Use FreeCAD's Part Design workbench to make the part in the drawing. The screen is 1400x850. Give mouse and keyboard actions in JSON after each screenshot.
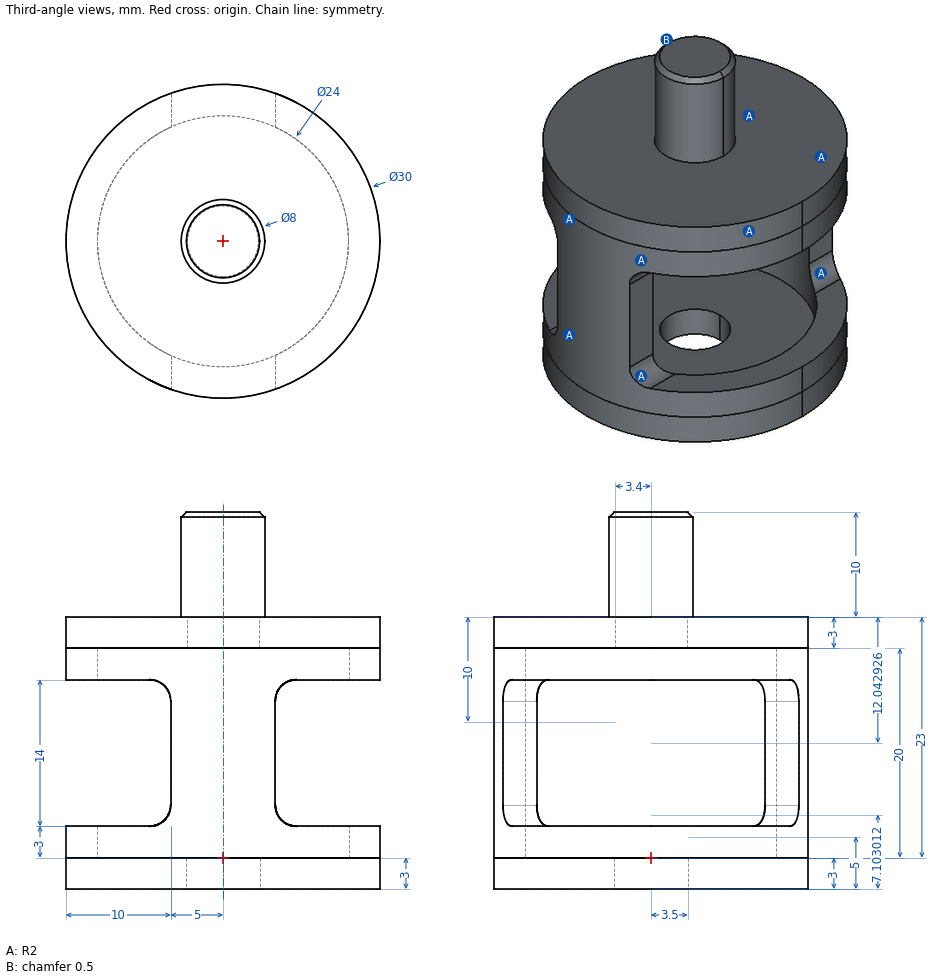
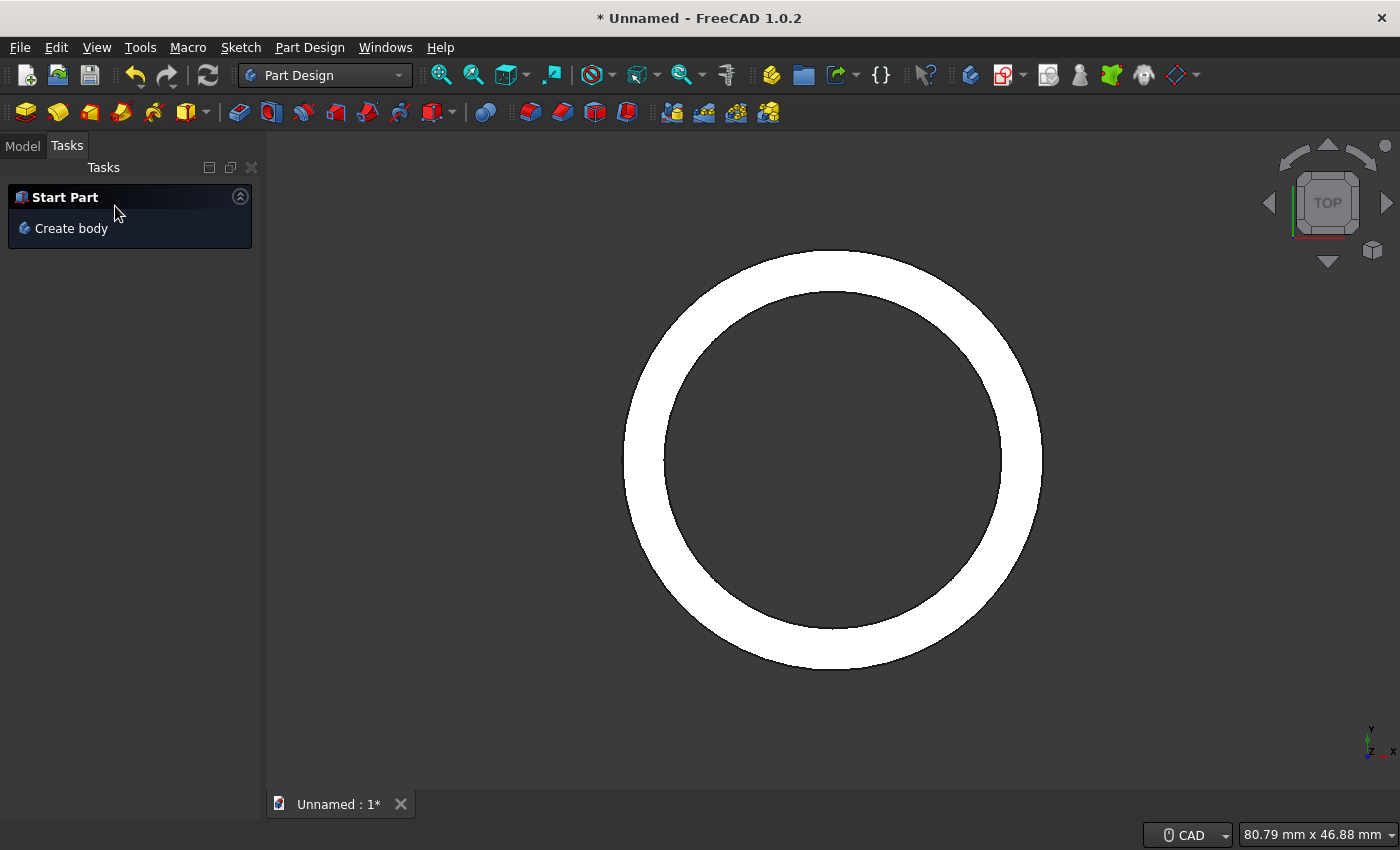
{"action": "key", "text": "1"}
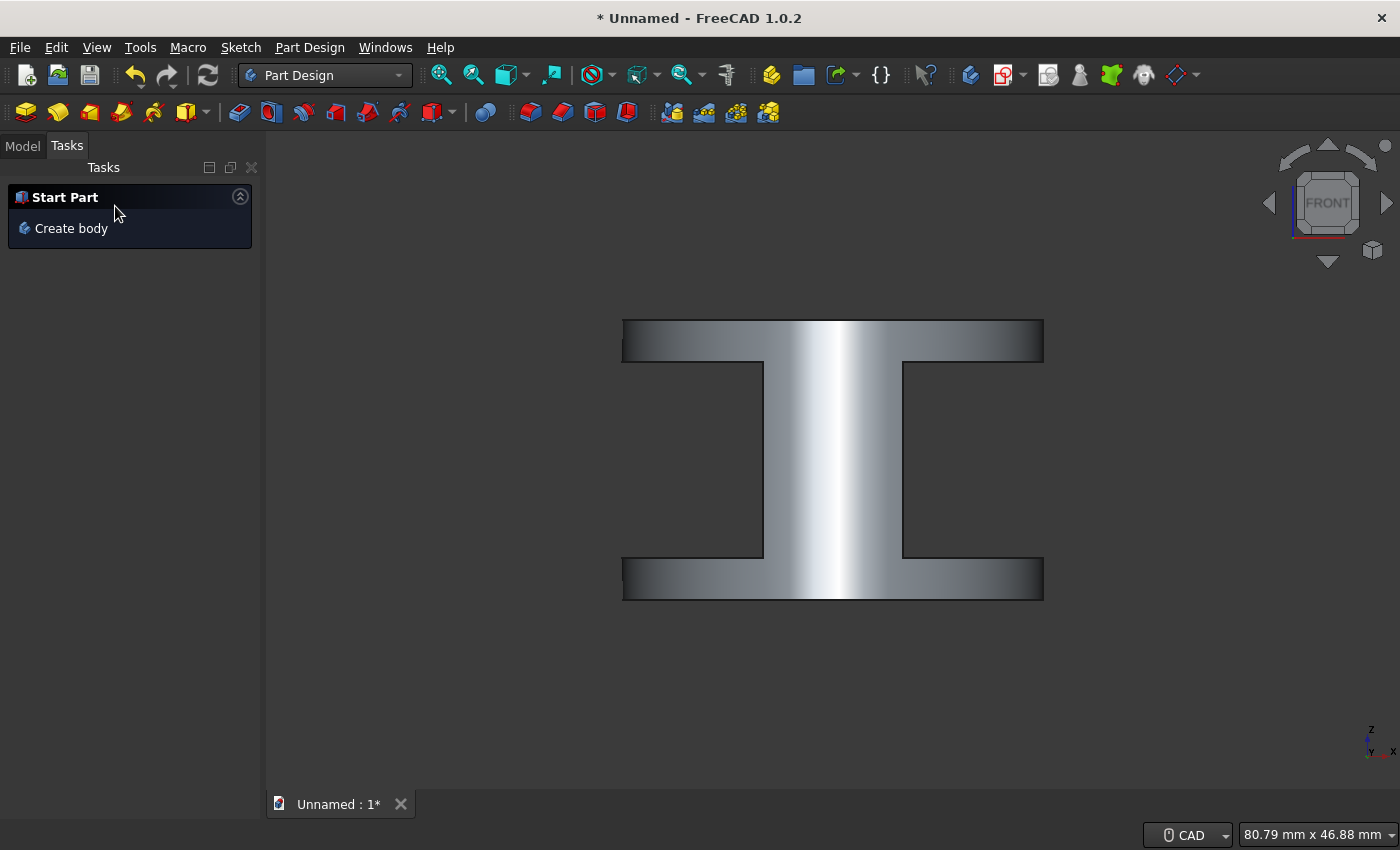
{"action": "key", "text": "v f"}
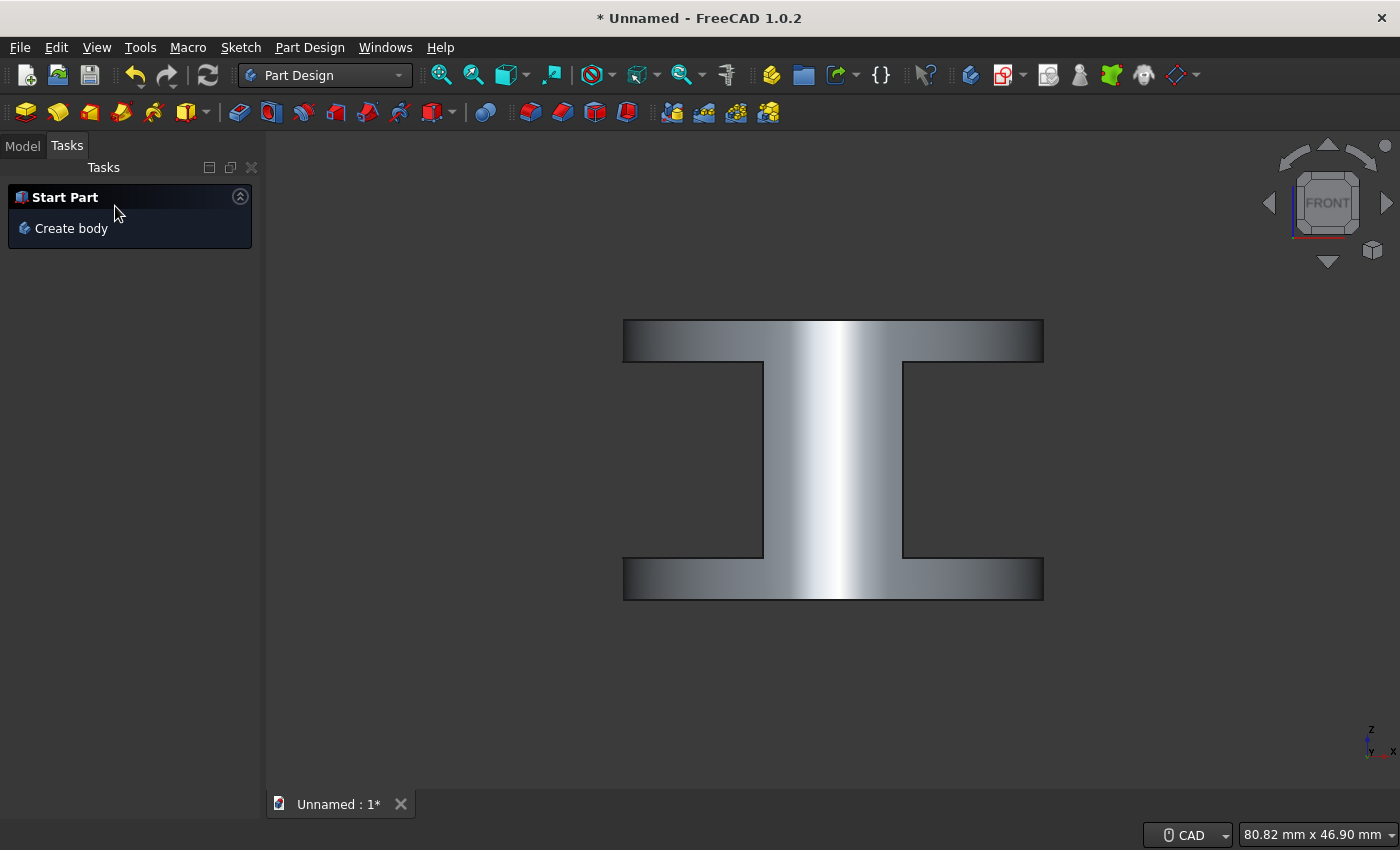
{"action": "key", "text": "3"}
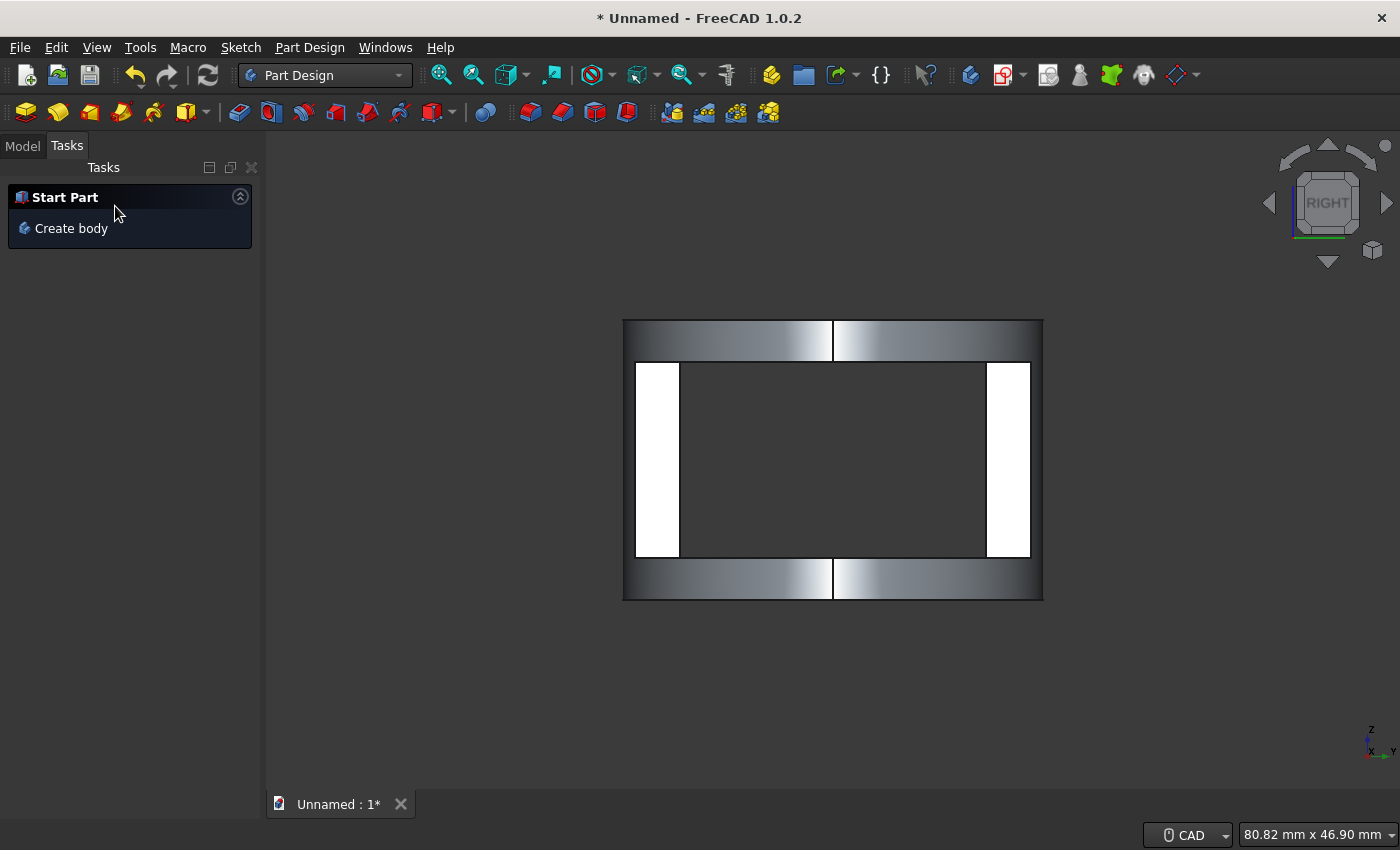
{"action": "key", "text": "v f"}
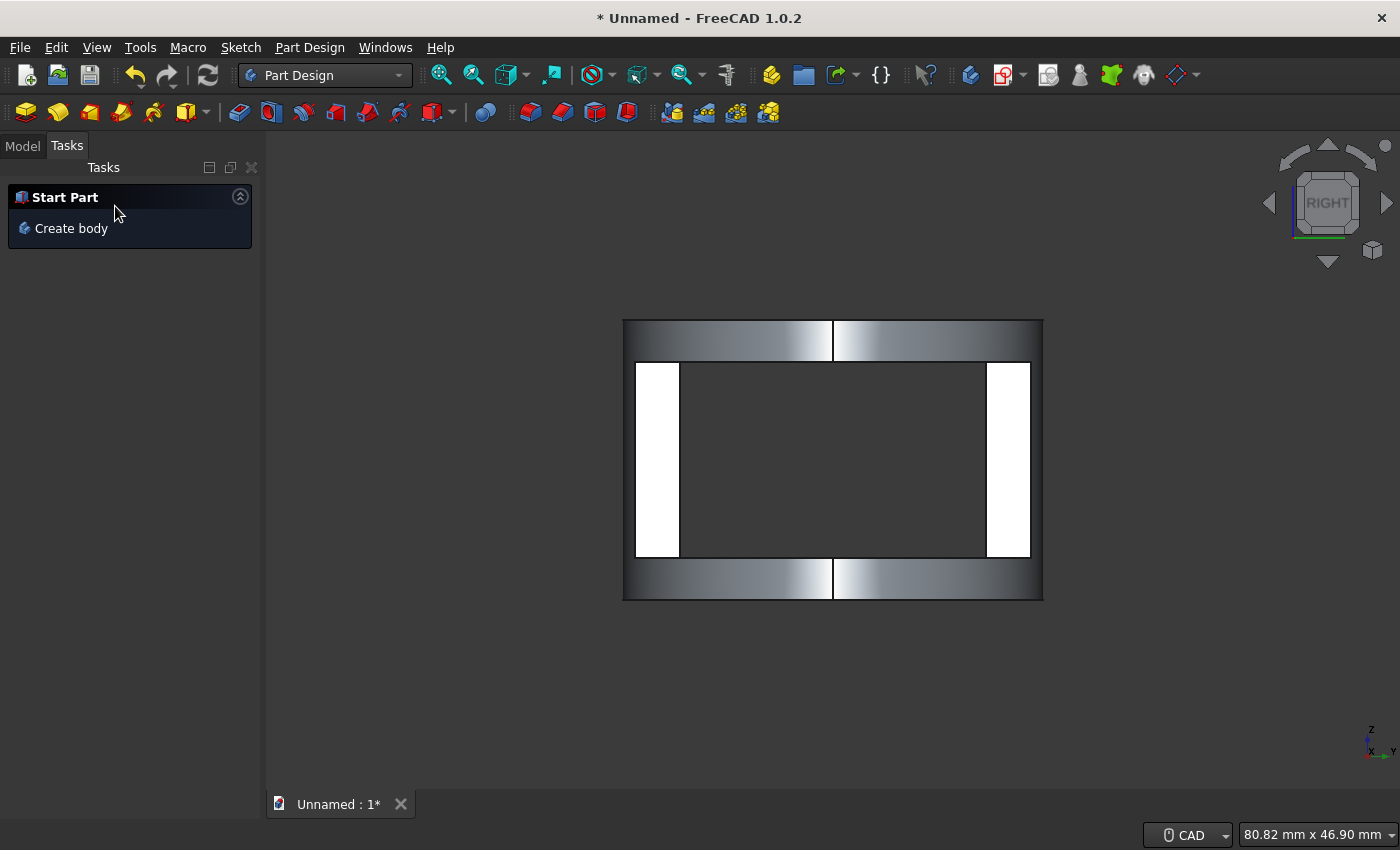
{"action": "key", "text": "5"}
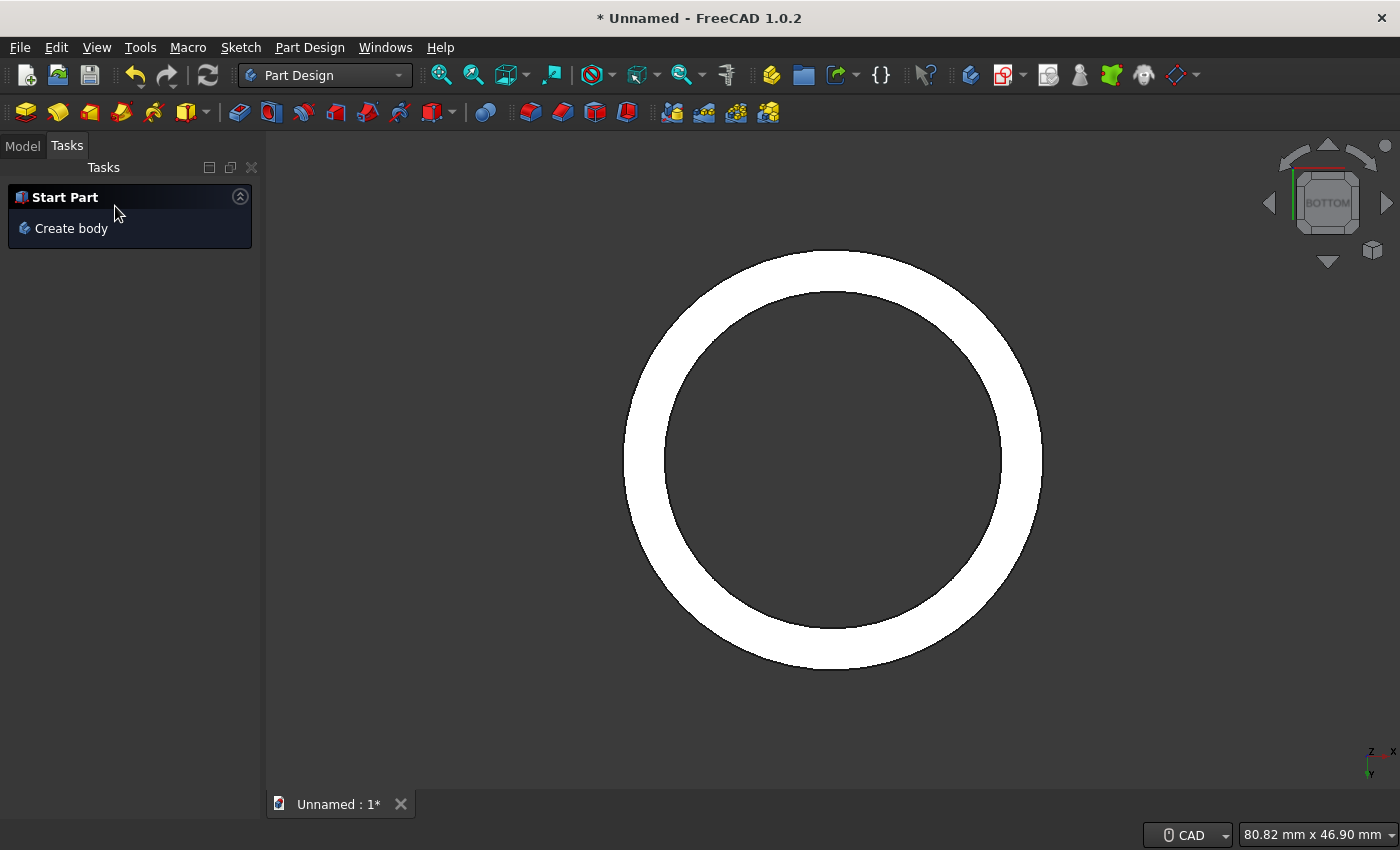
{"action": "key", "text": "4"}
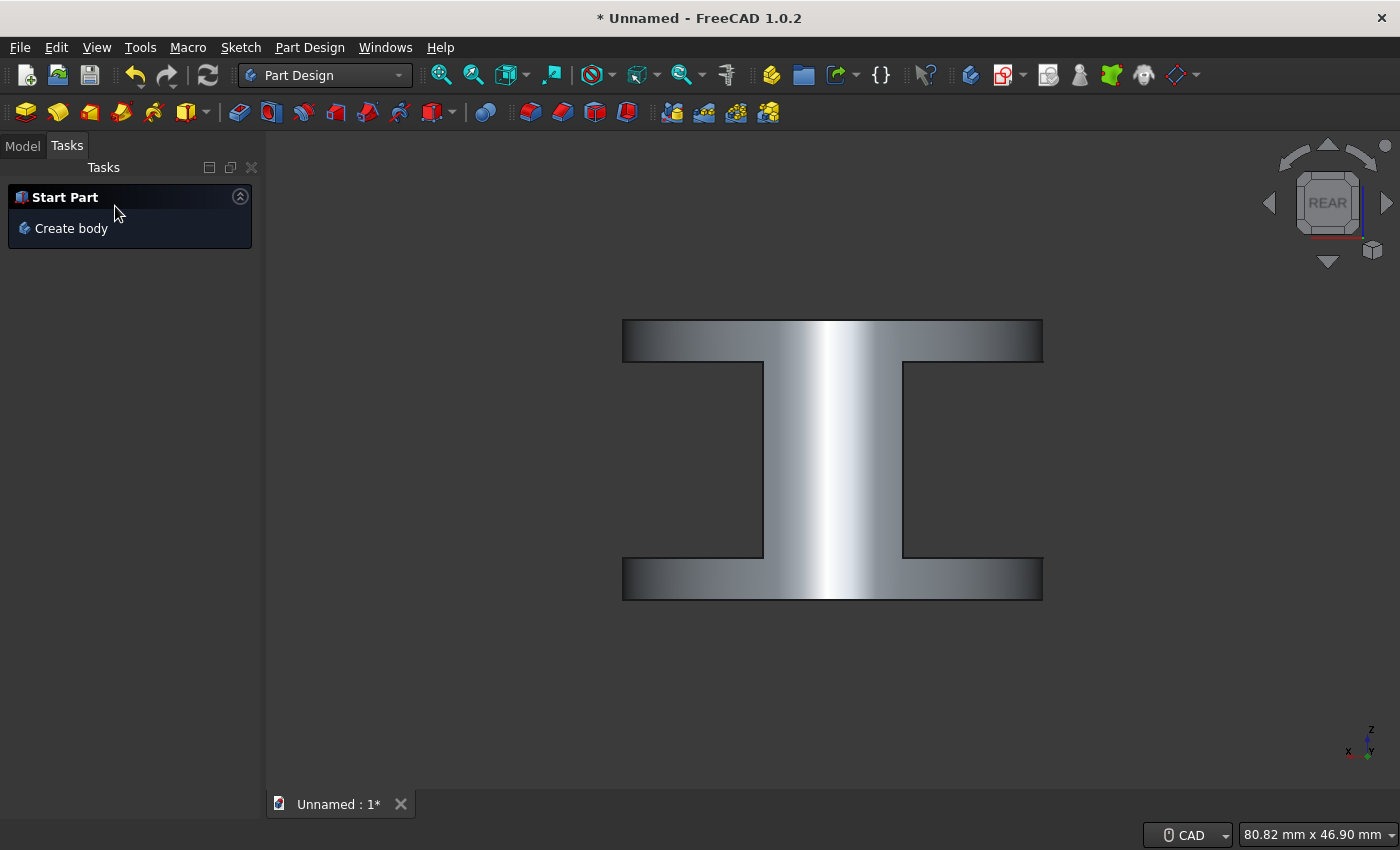
{"action": "left_click", "coordinate": [442, 76]}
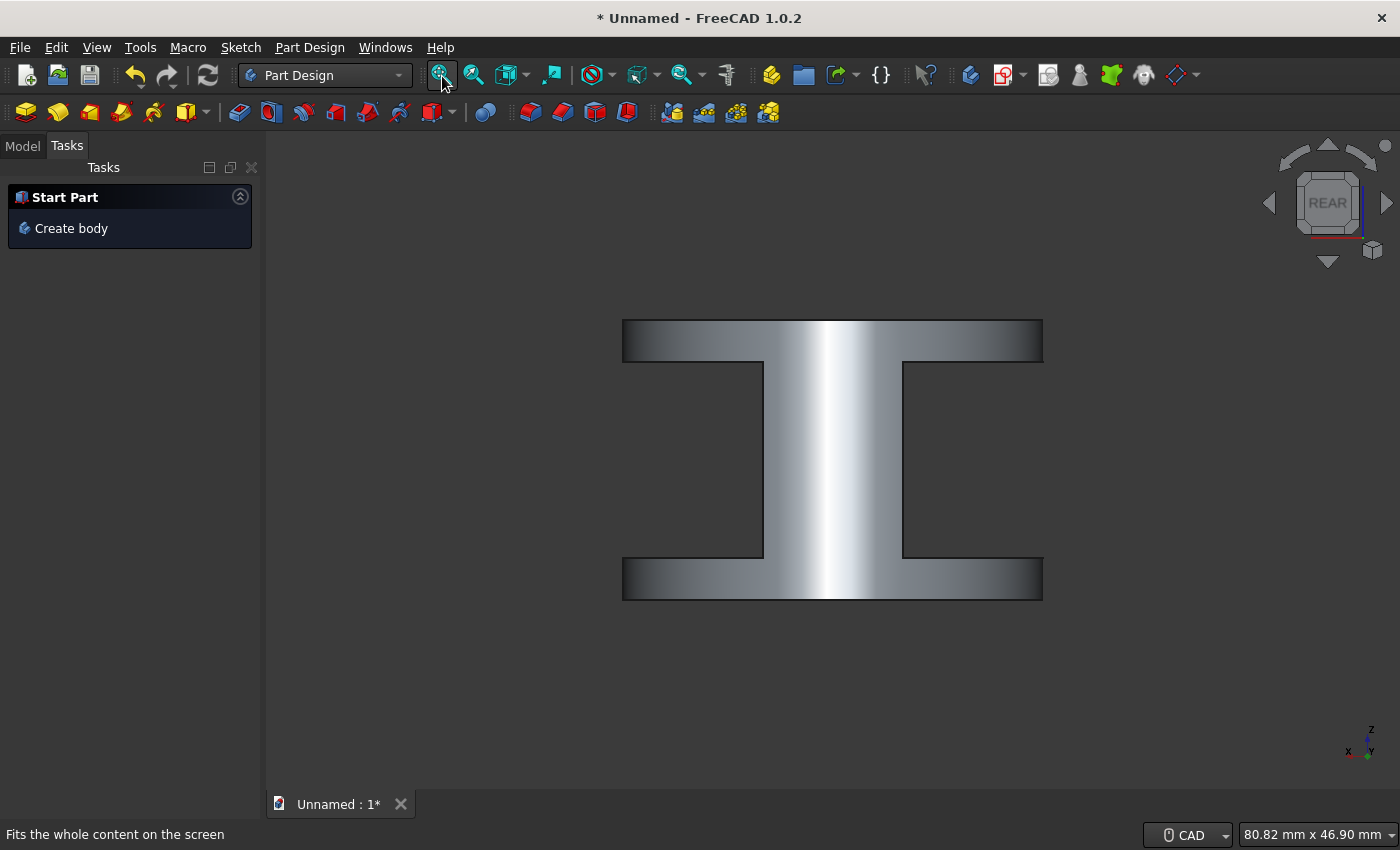
{"action": "key", "text": "6"}